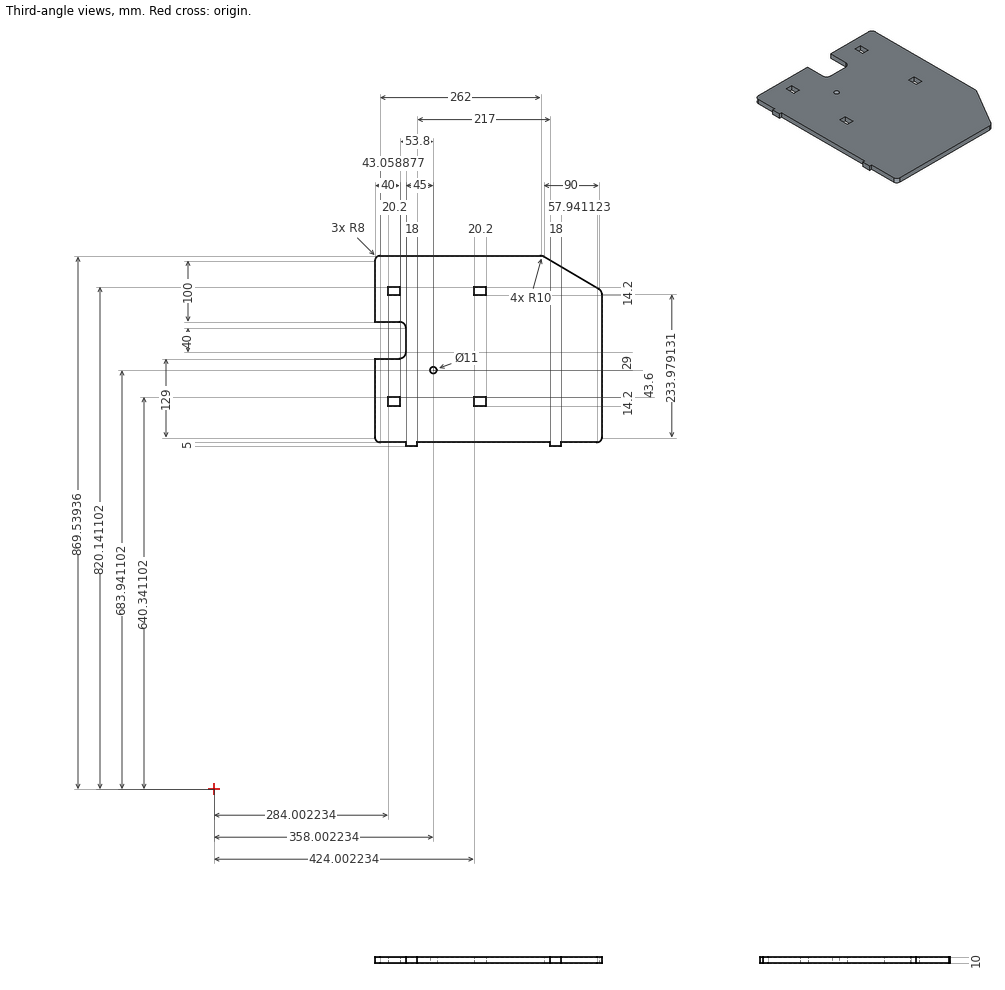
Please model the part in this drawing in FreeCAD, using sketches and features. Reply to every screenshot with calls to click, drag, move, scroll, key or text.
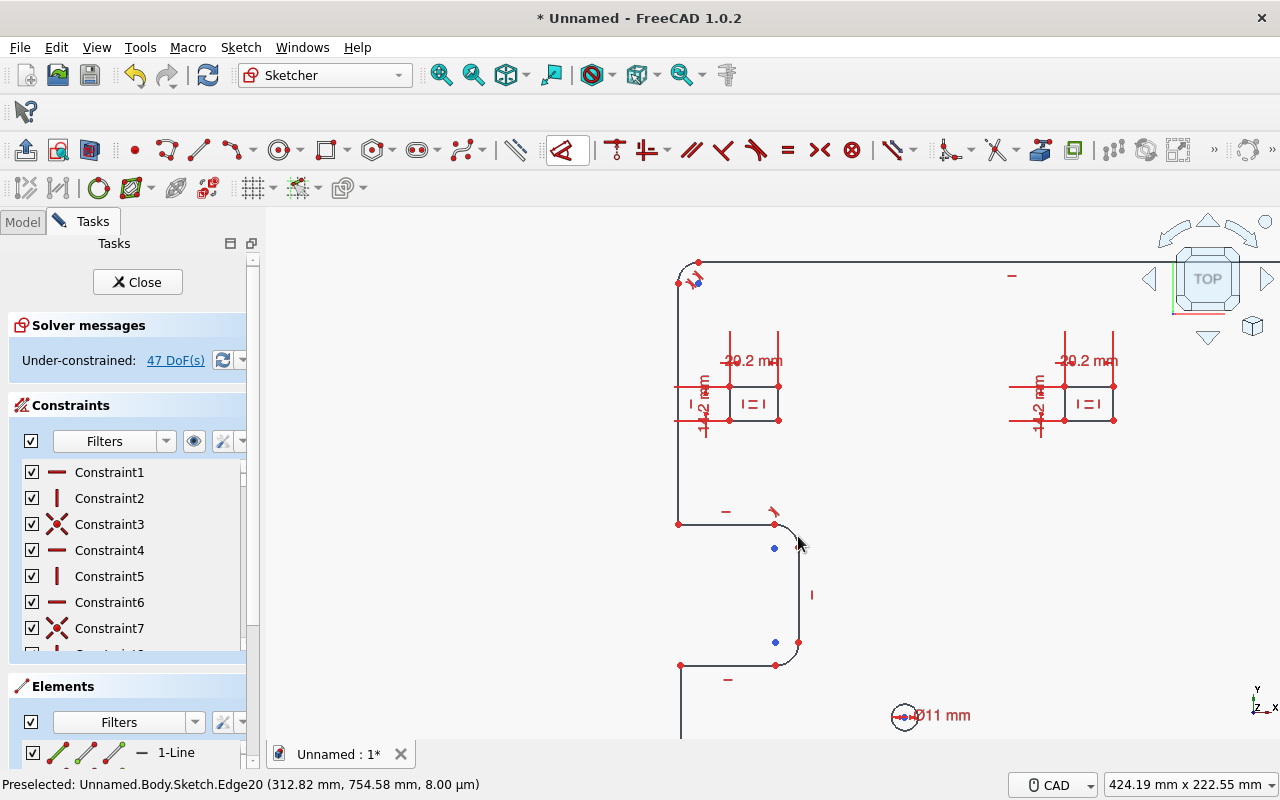
click(799, 576)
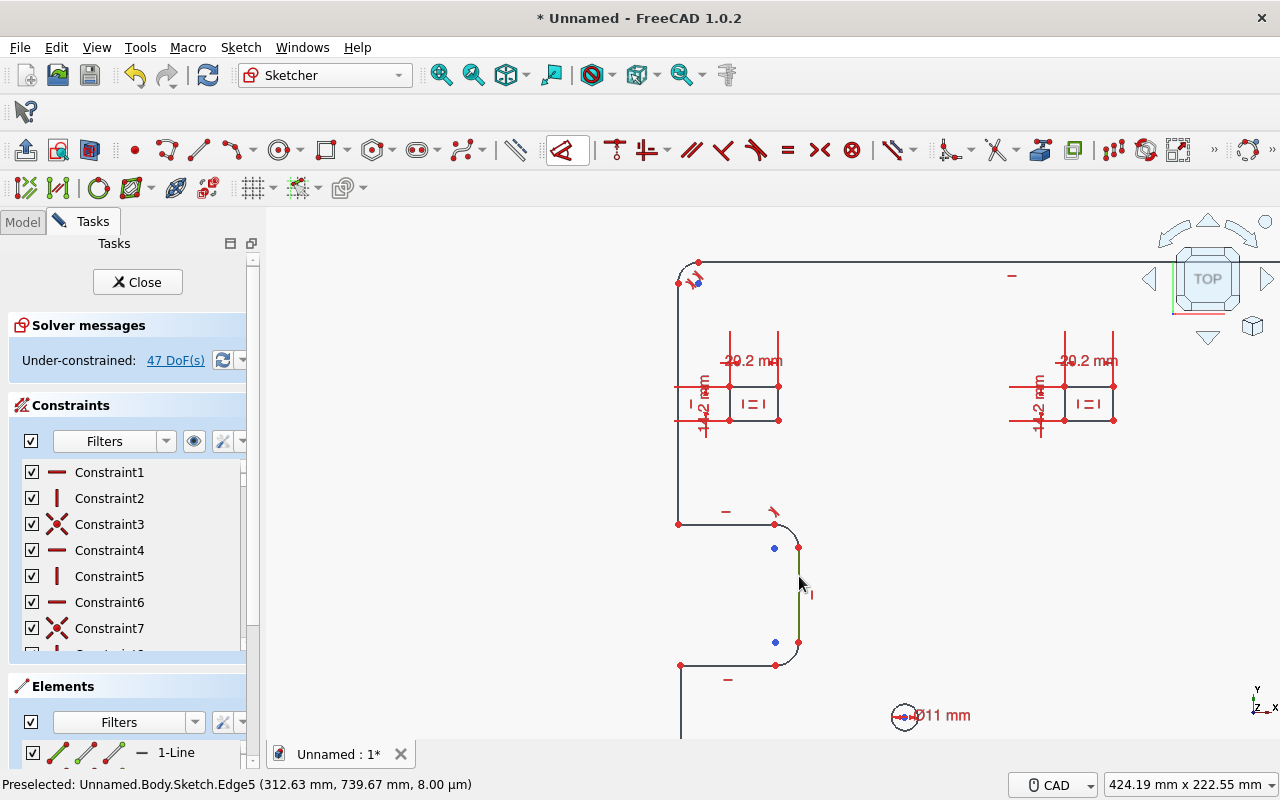
scroll(796, 537, up, 2)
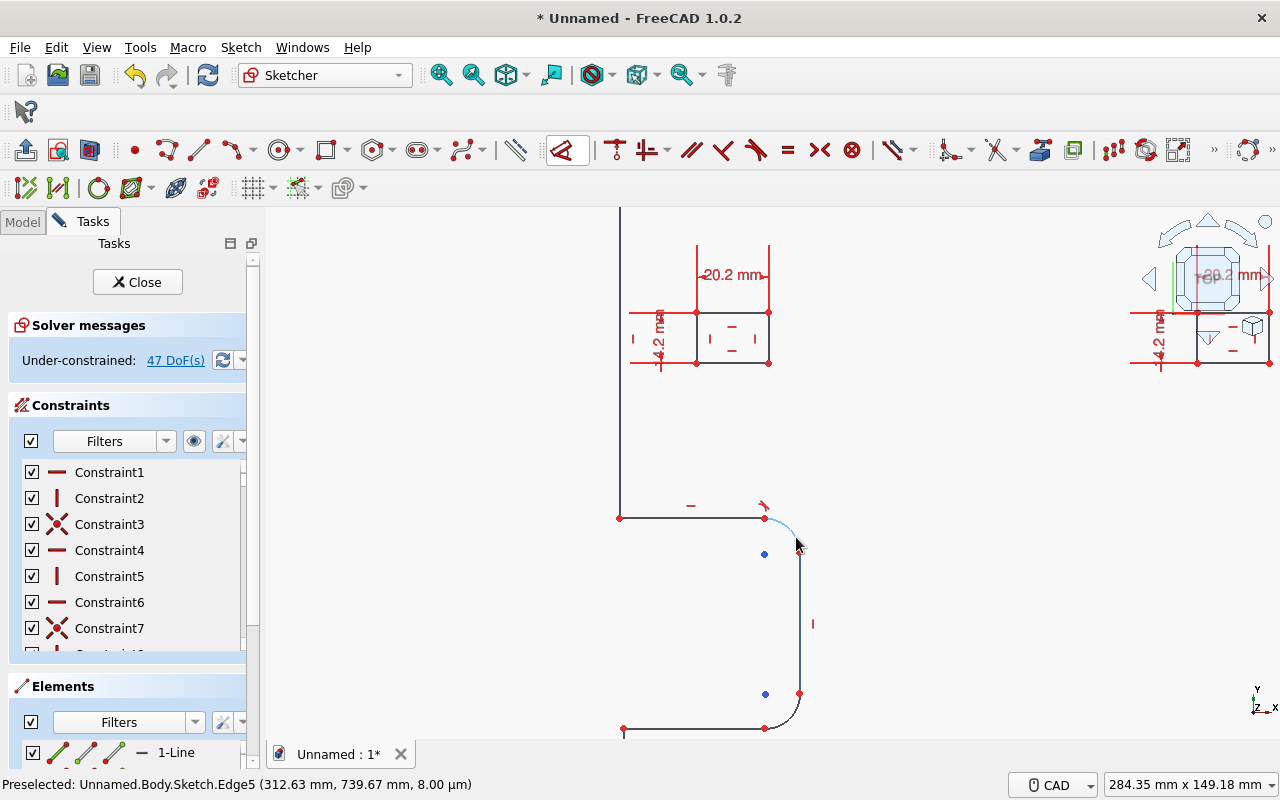
click(796, 537)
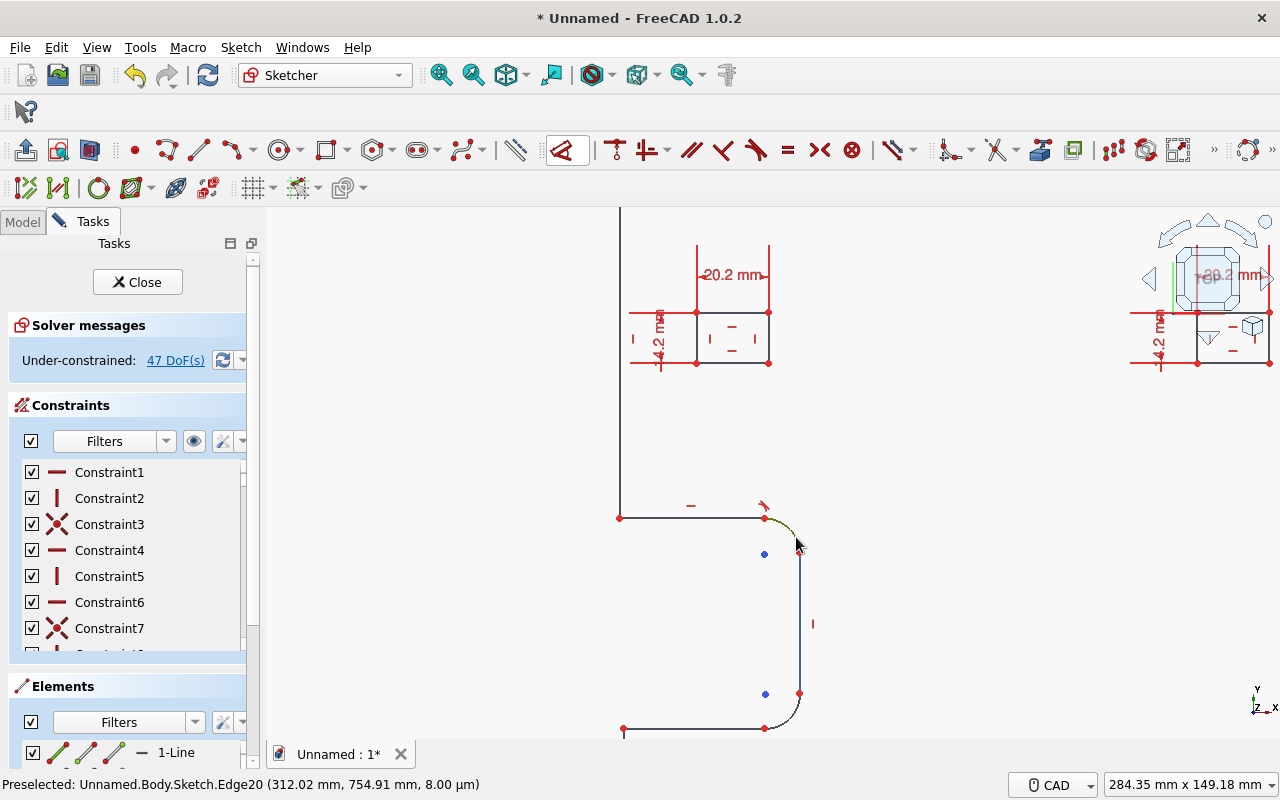
click(756, 150)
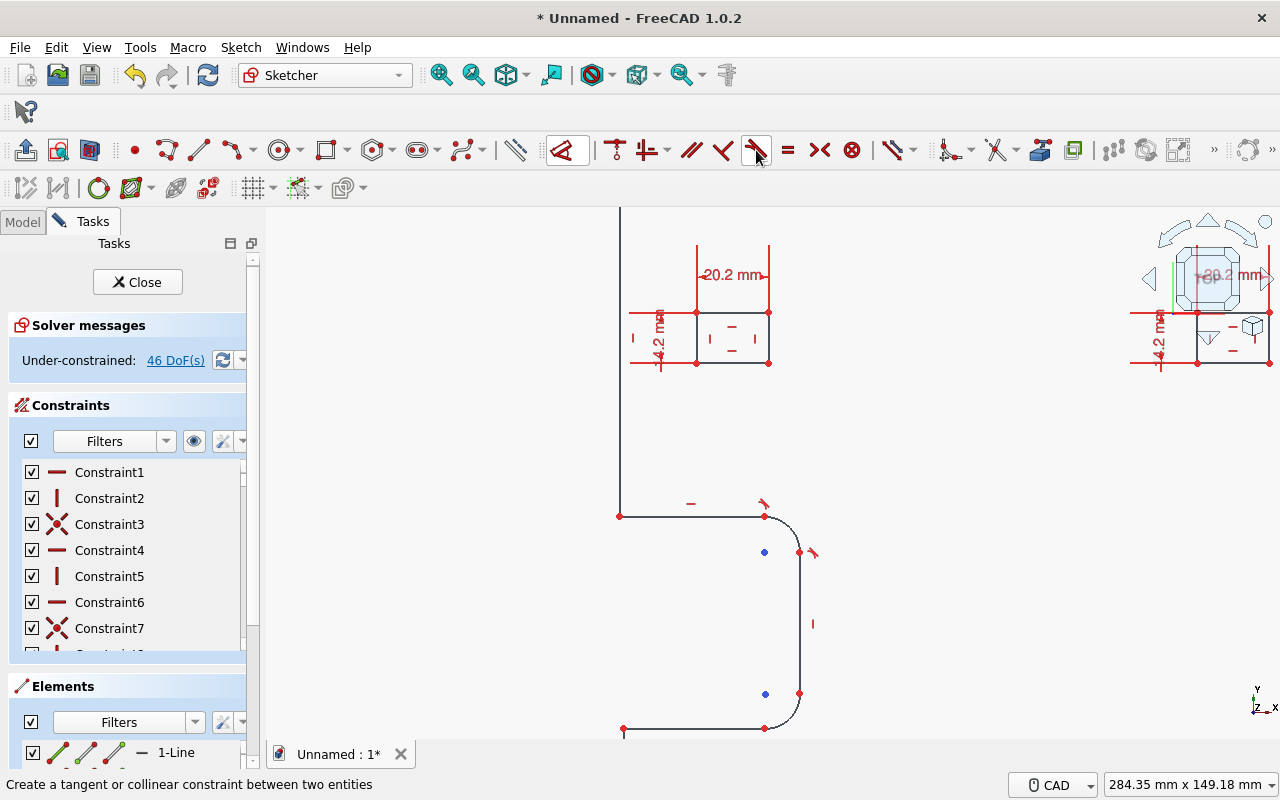
scroll(691, 322, down, 11)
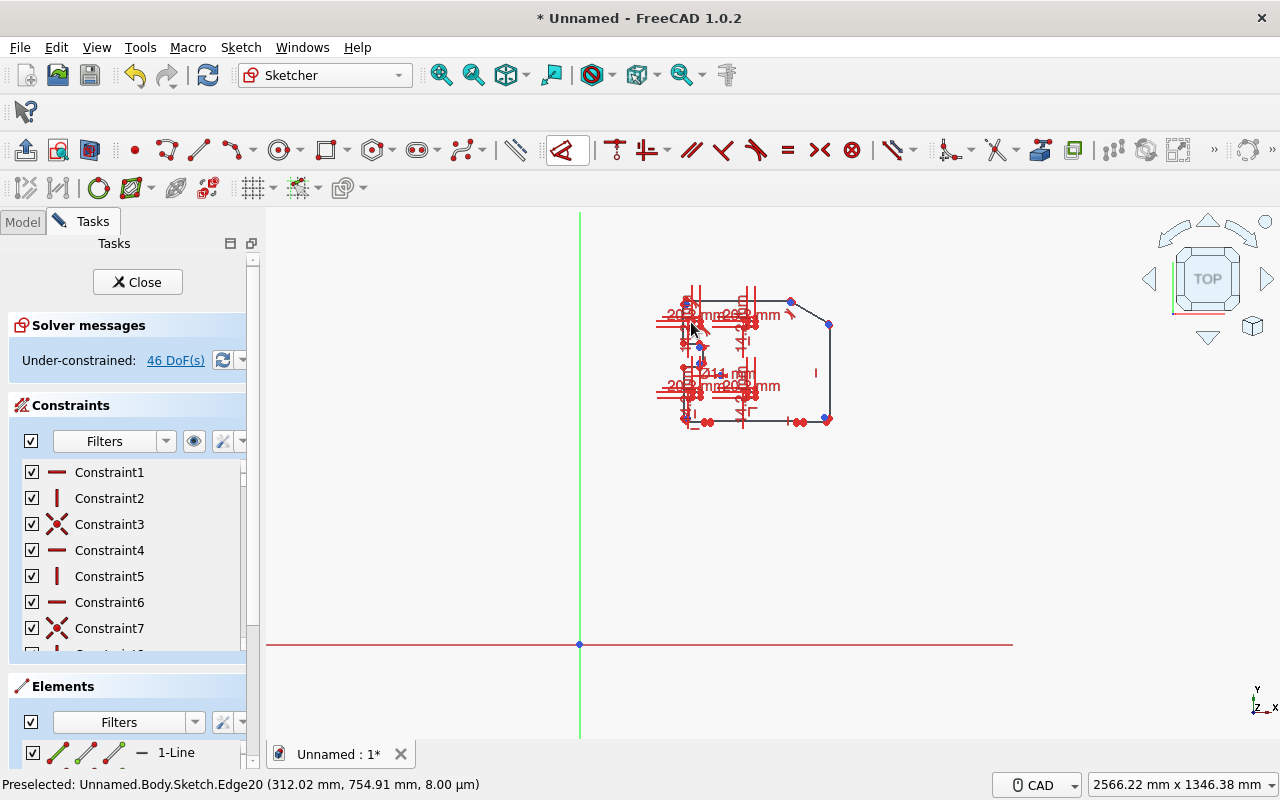
scroll(703, 352, up, 6)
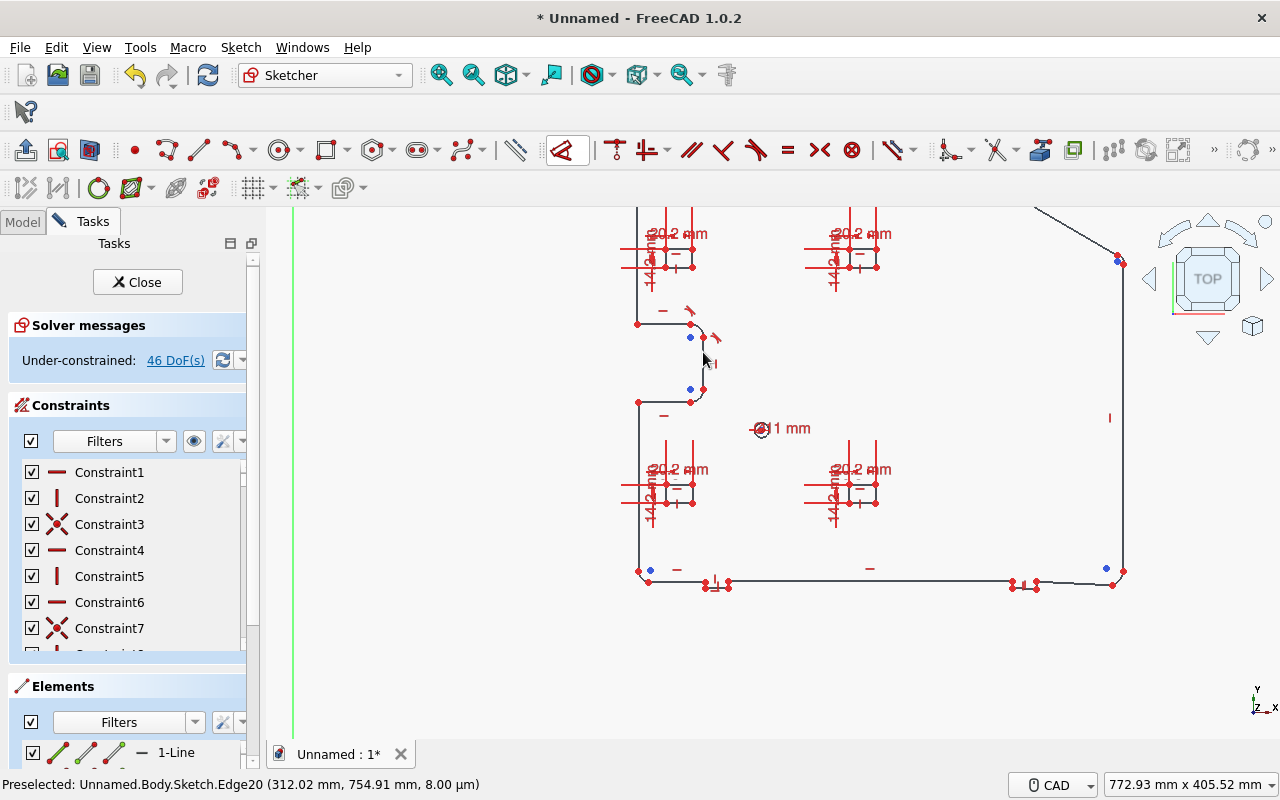
click(703, 353)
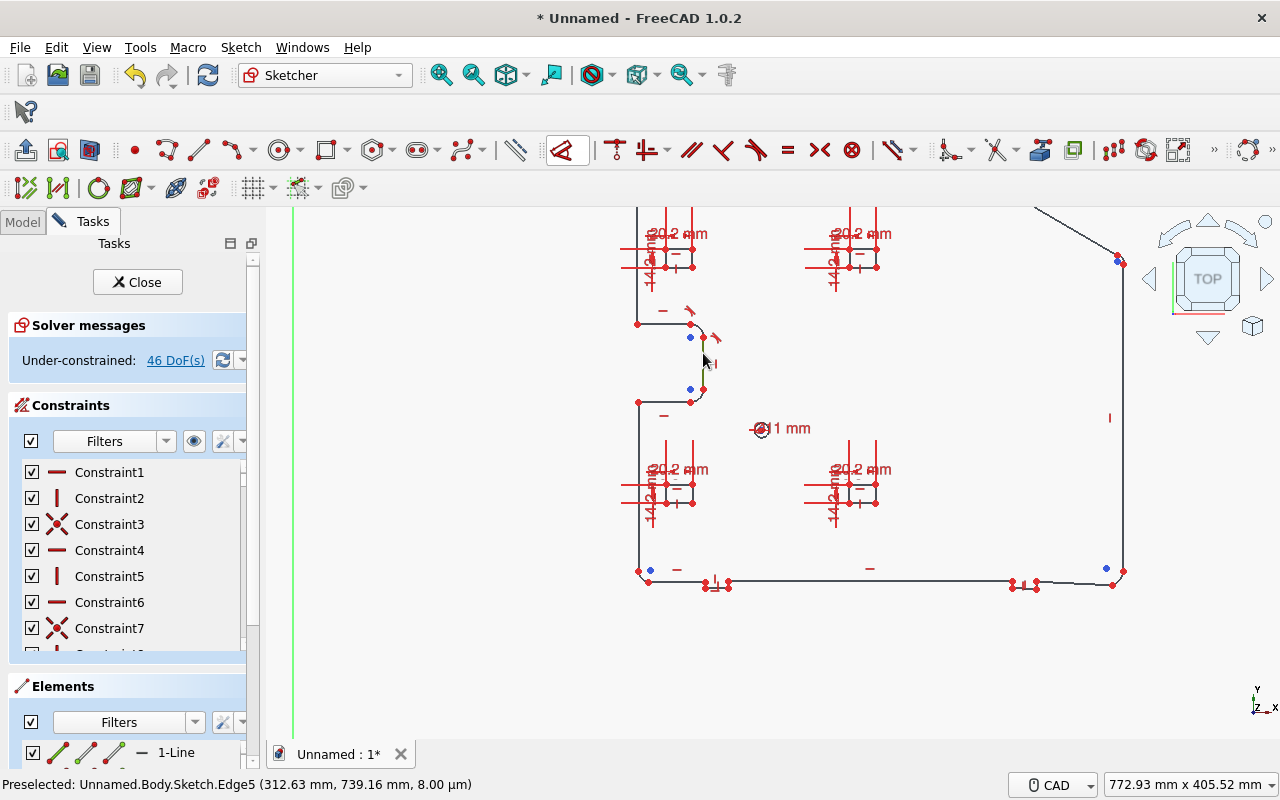
scroll(700, 398, up, 2)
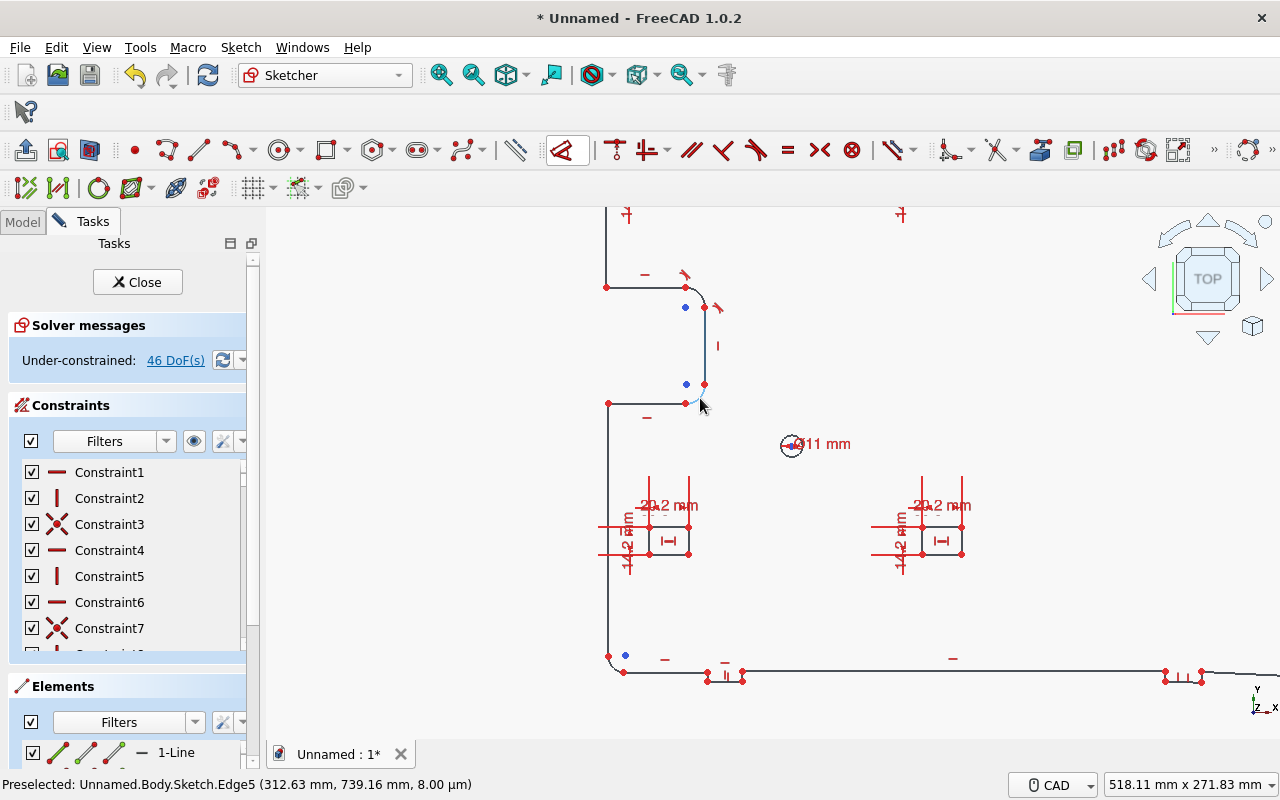
click(699, 398)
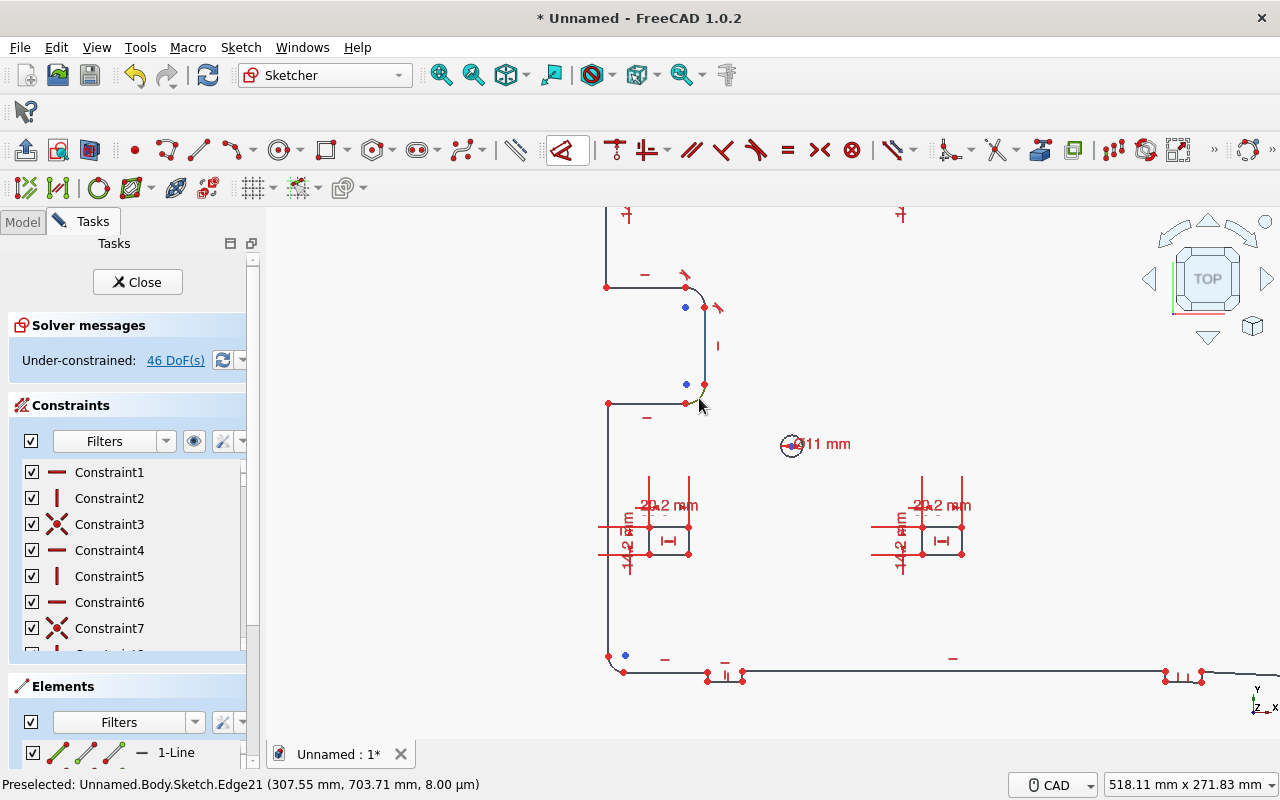
click(756, 150)